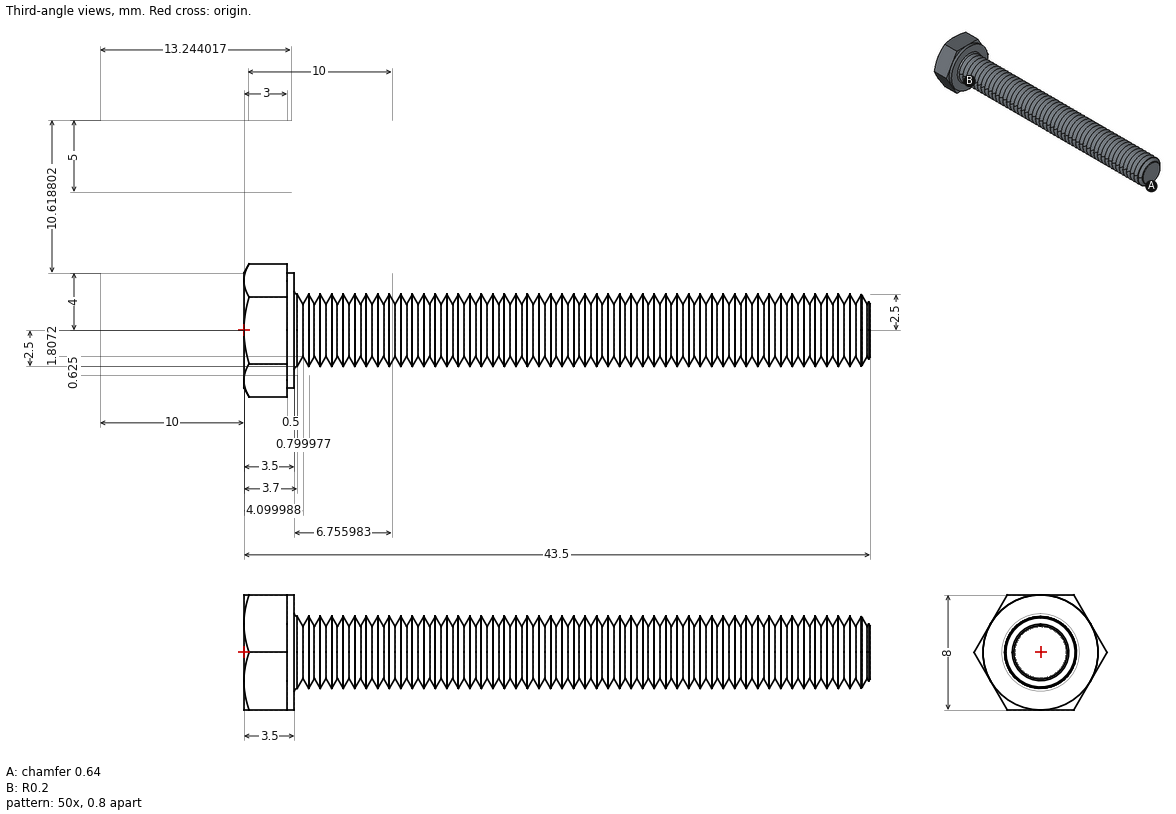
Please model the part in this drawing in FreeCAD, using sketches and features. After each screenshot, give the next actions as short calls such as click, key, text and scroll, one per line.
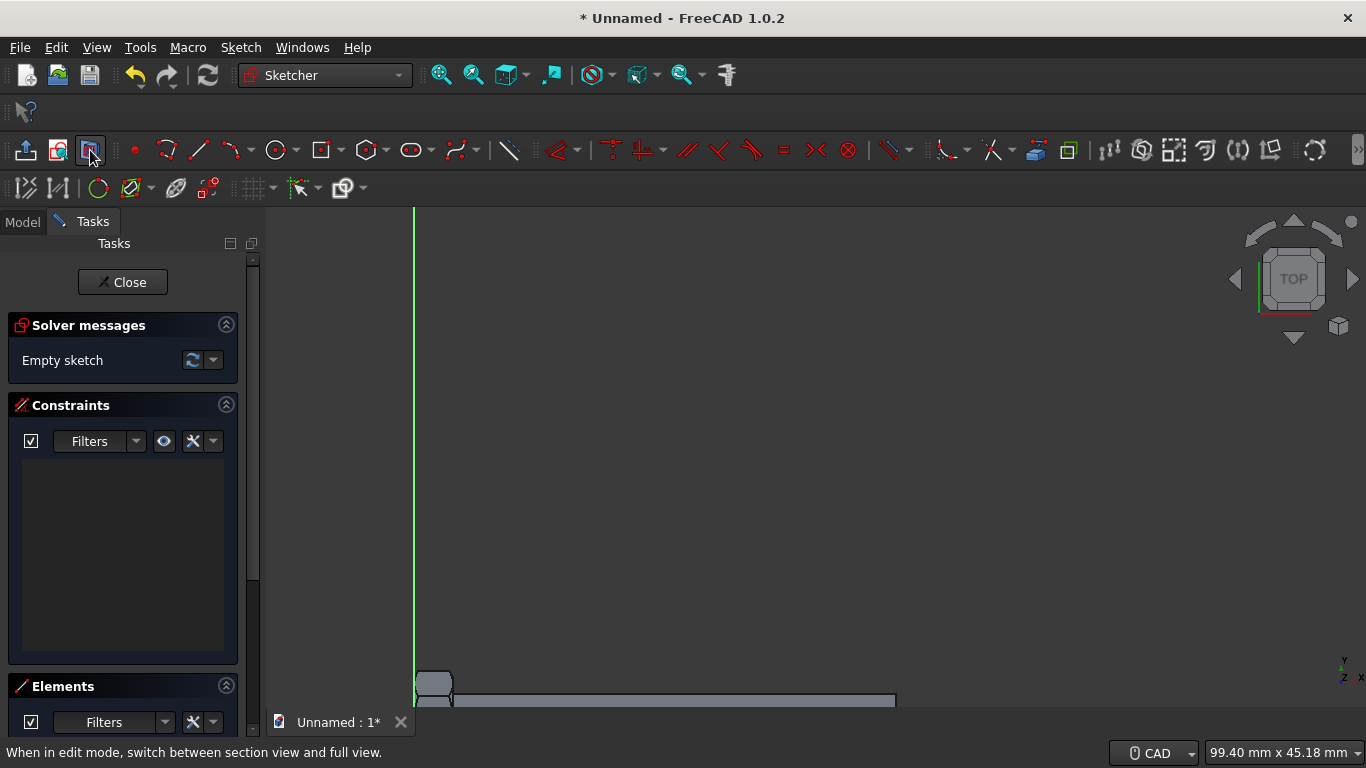
scroll(748, 457, down, 5)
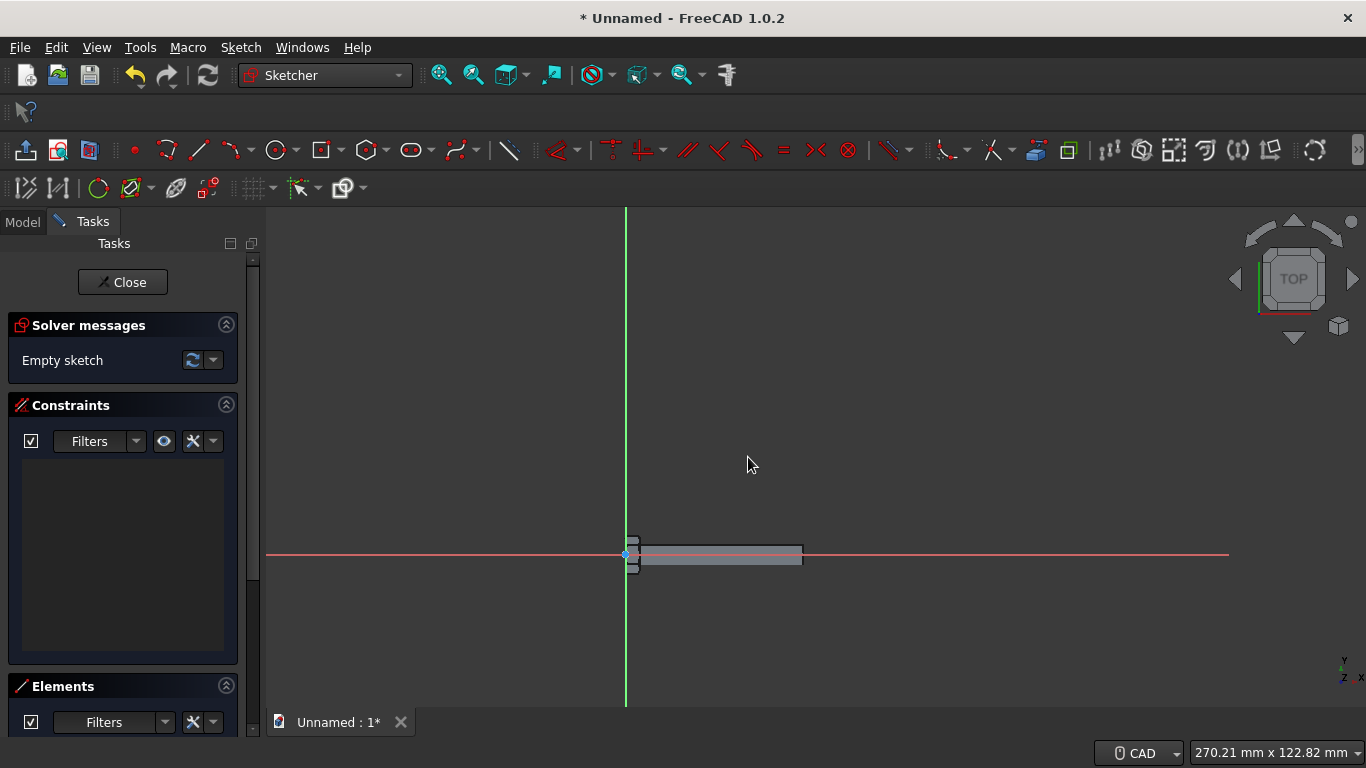
scroll(604, 542, up, 8)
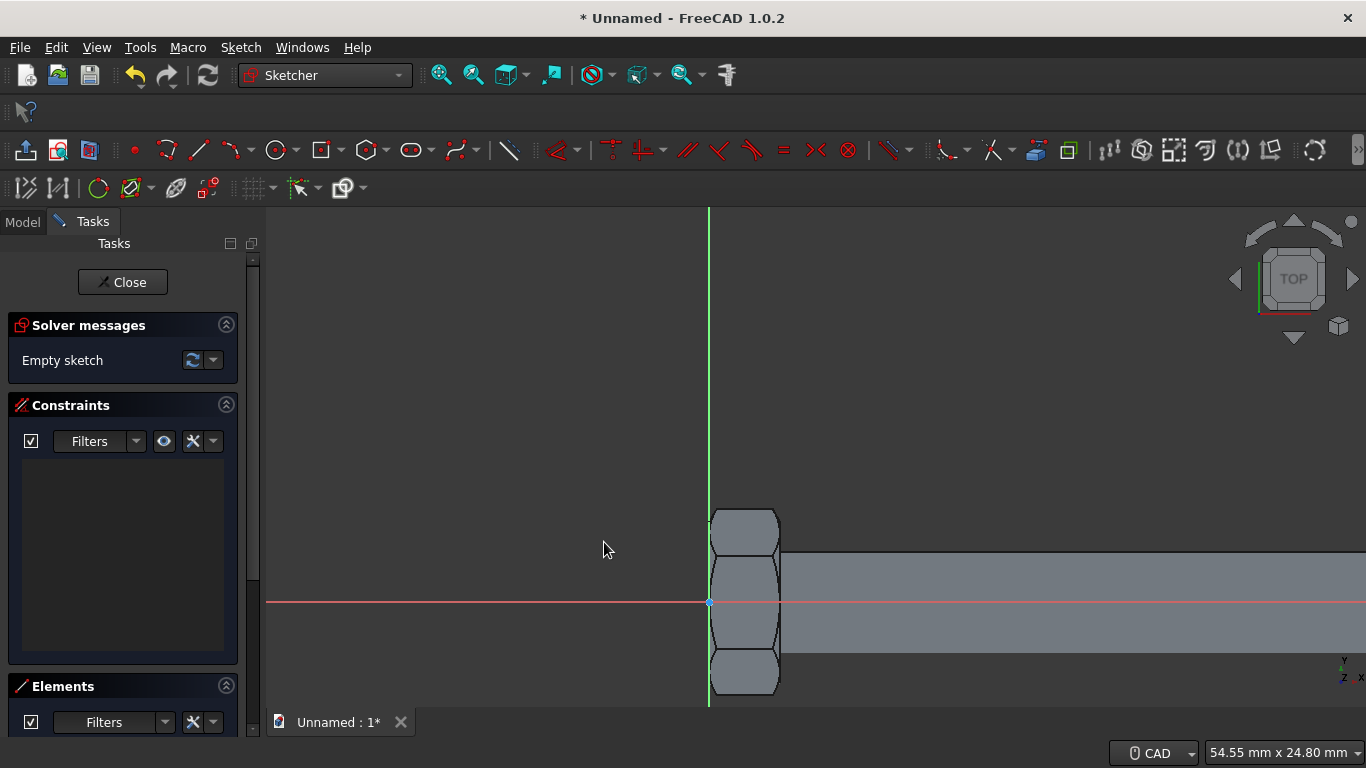
key(g)
key(r)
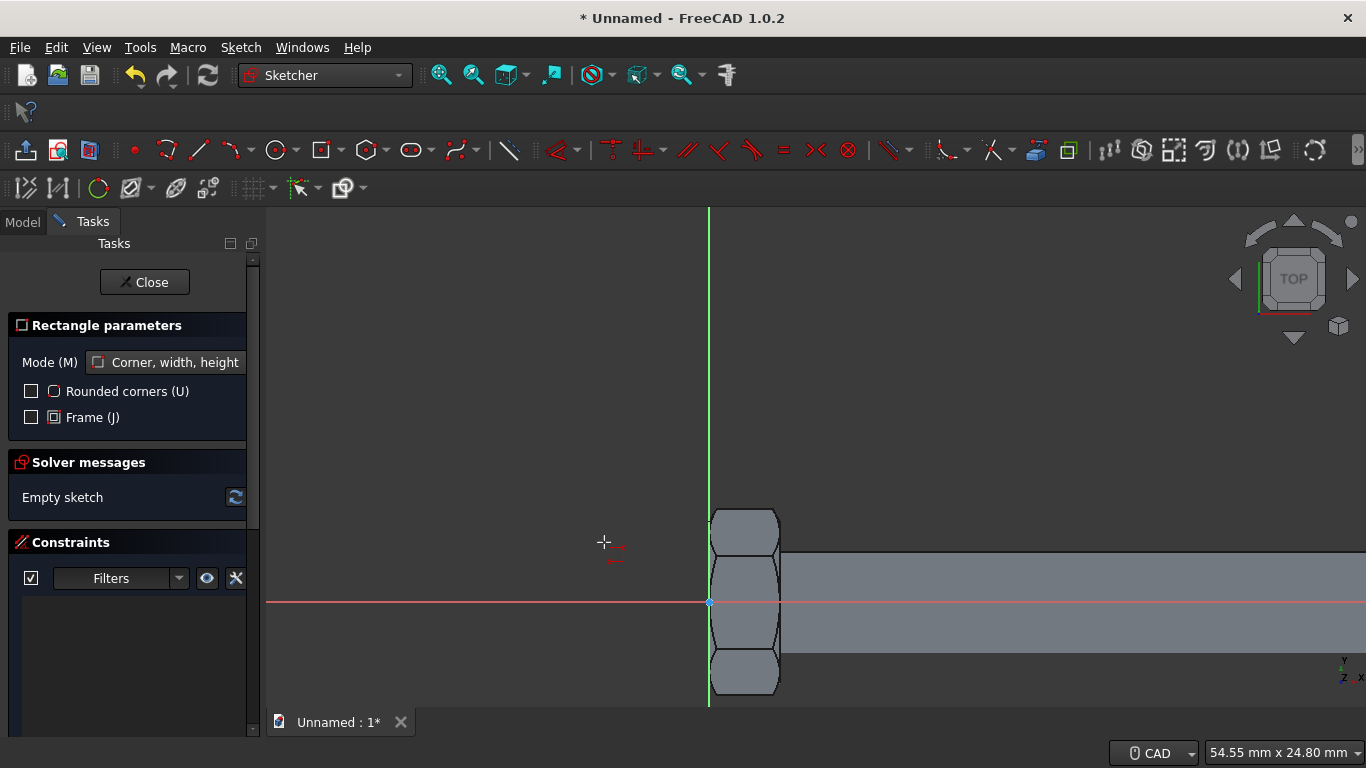
scroll(770, 308, up, 3)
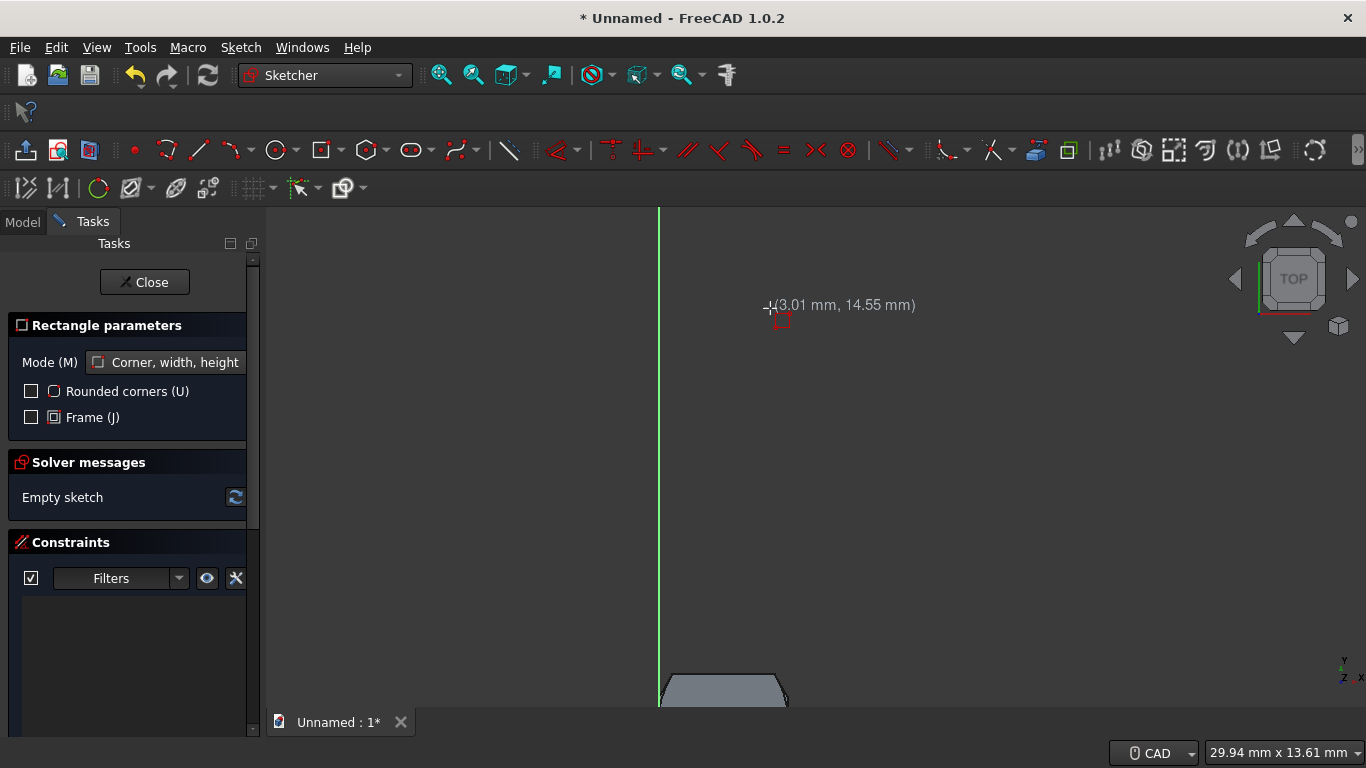
click(769, 307)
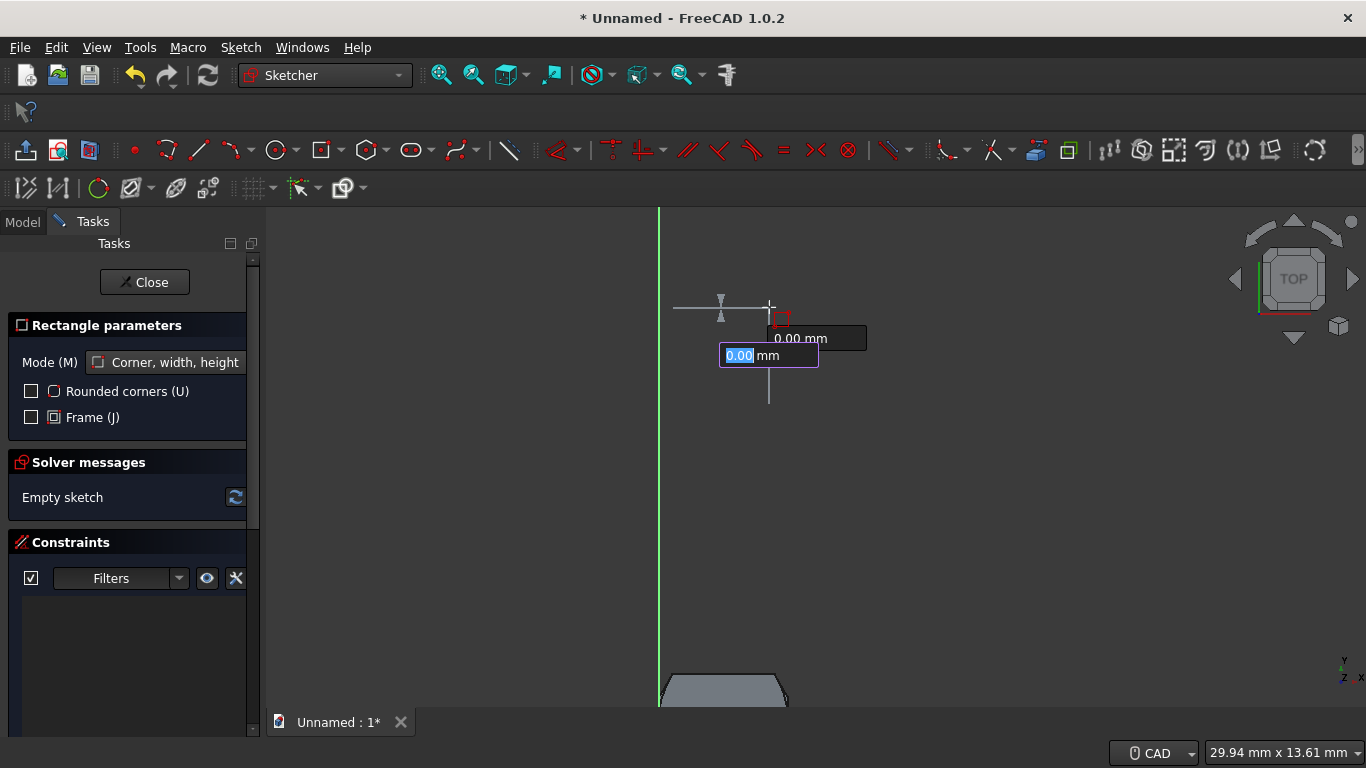
scroll(777, 313, down, 3)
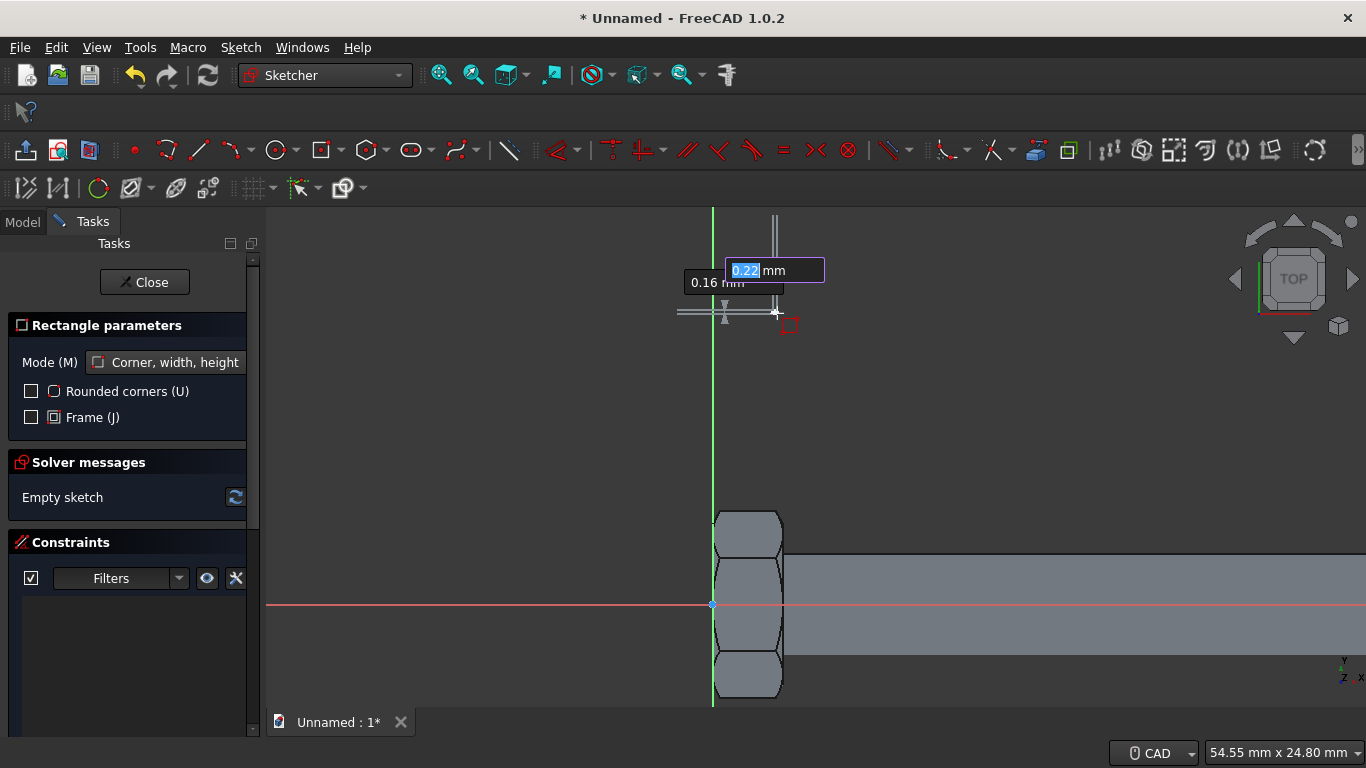
click(783, 524)
key(Escape)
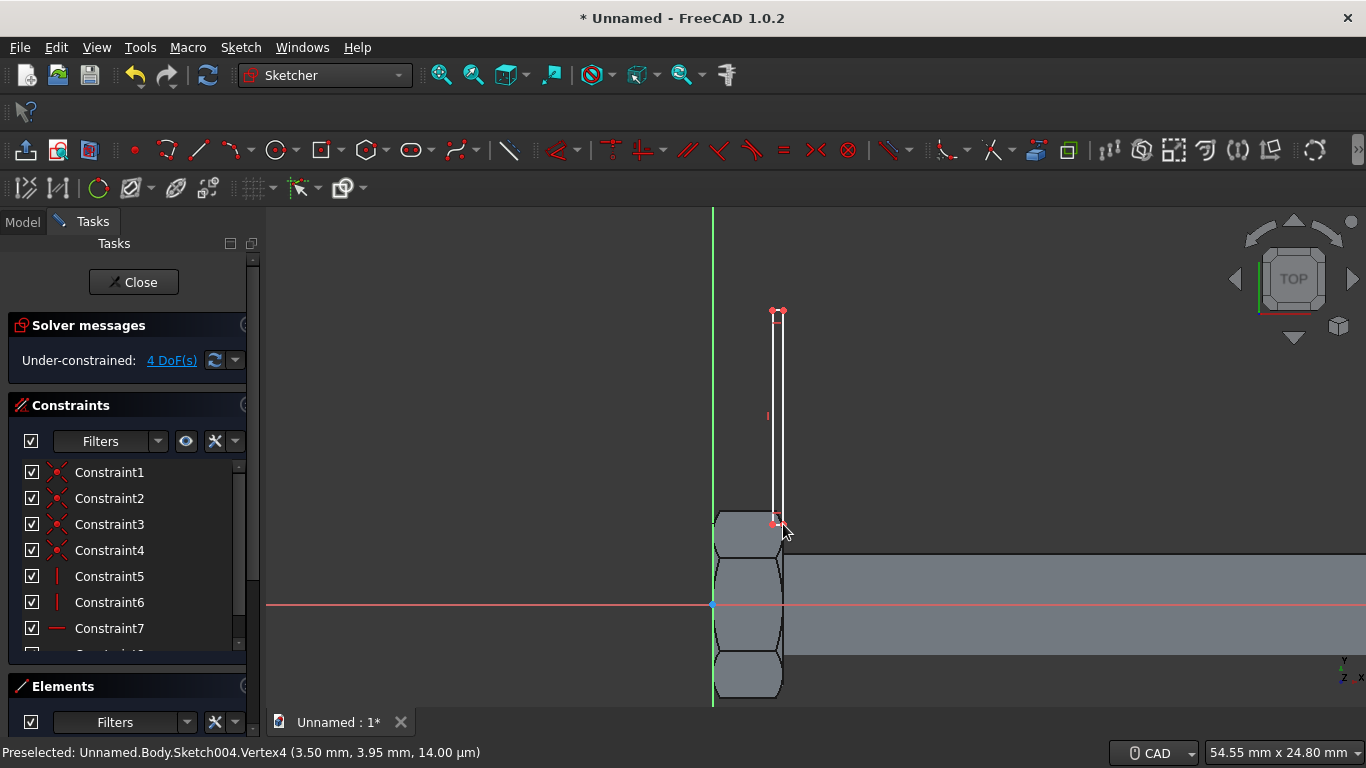
click(556, 150)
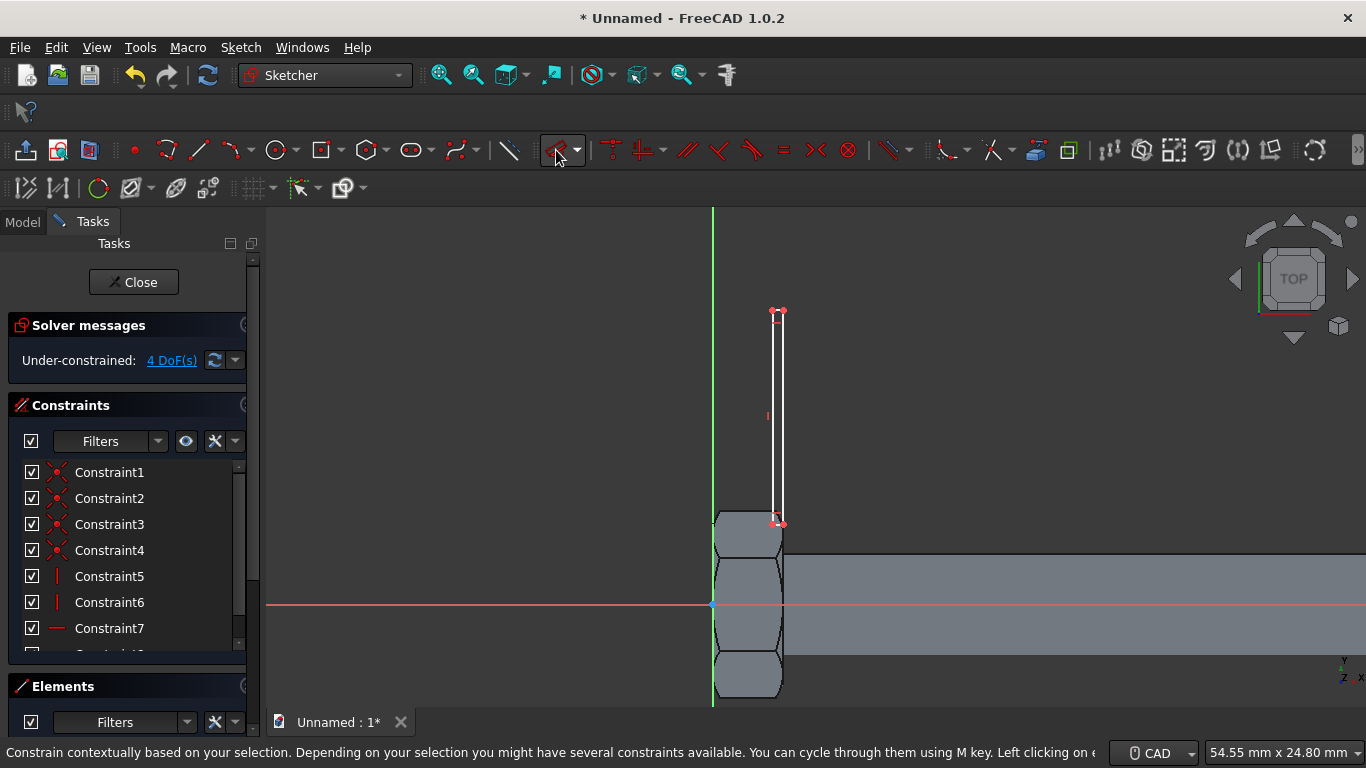
click(773, 310)
click(743, 639)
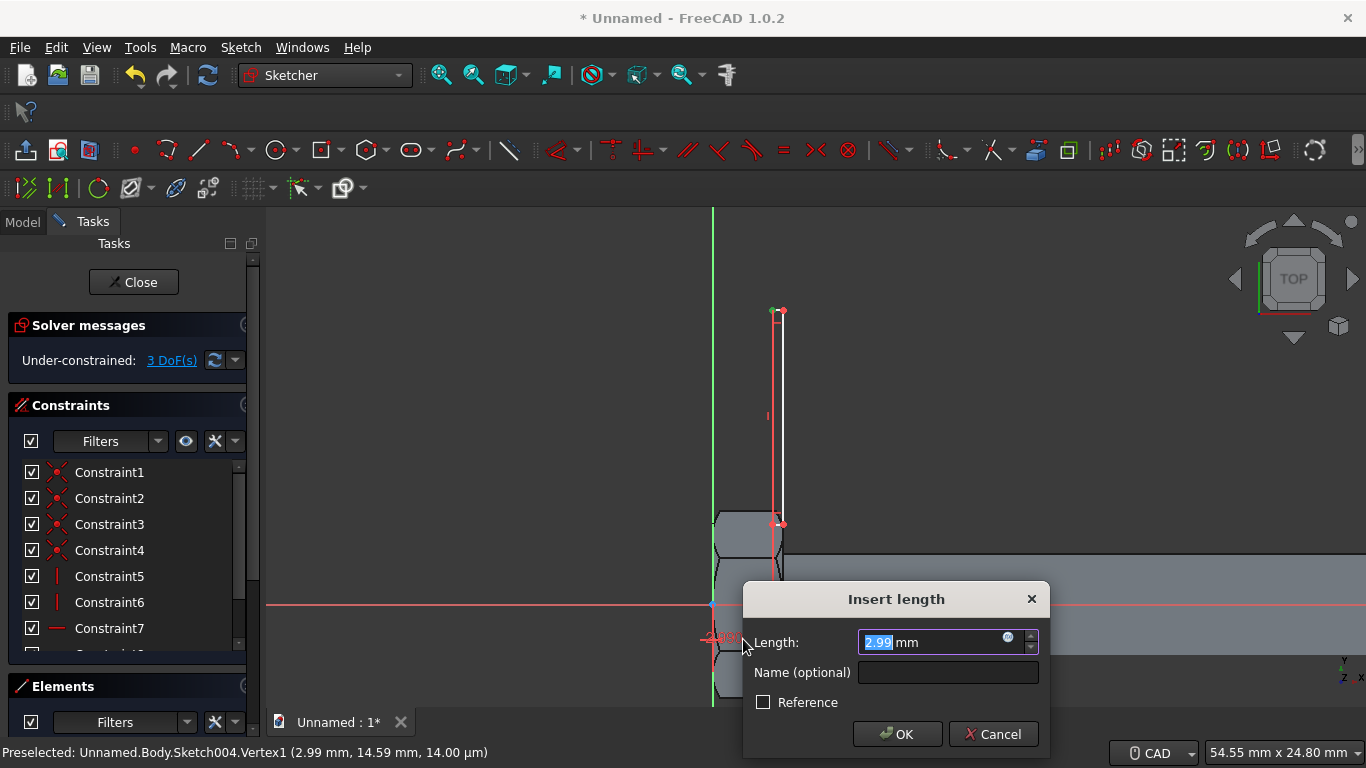
text(3)
key(Return)